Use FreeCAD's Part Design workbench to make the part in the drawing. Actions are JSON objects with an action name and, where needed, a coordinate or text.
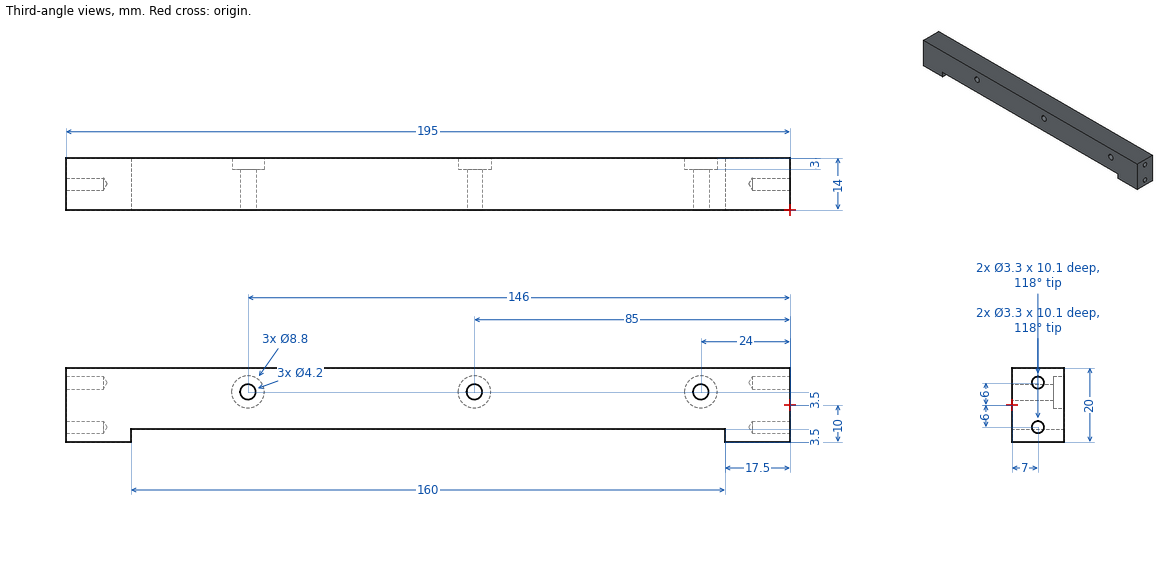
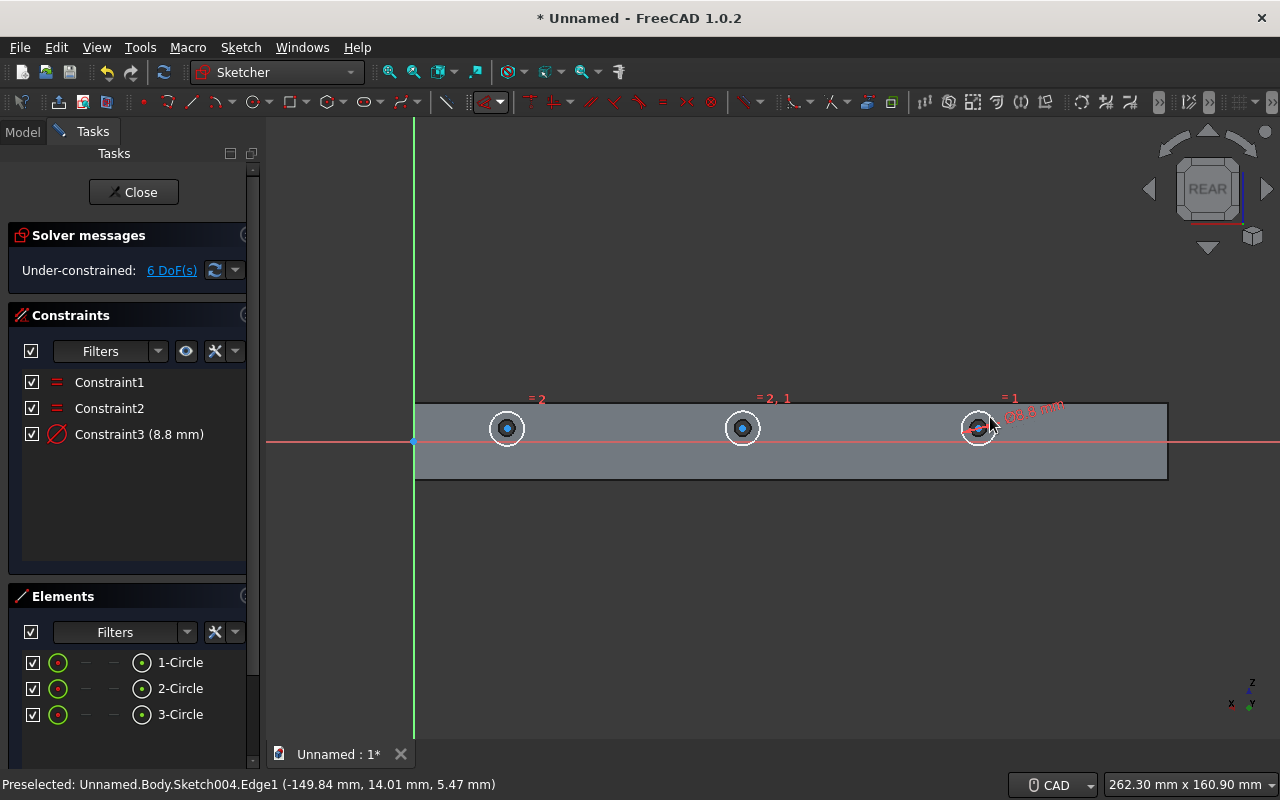
{"action": "left_click", "coordinate": [743, 428]}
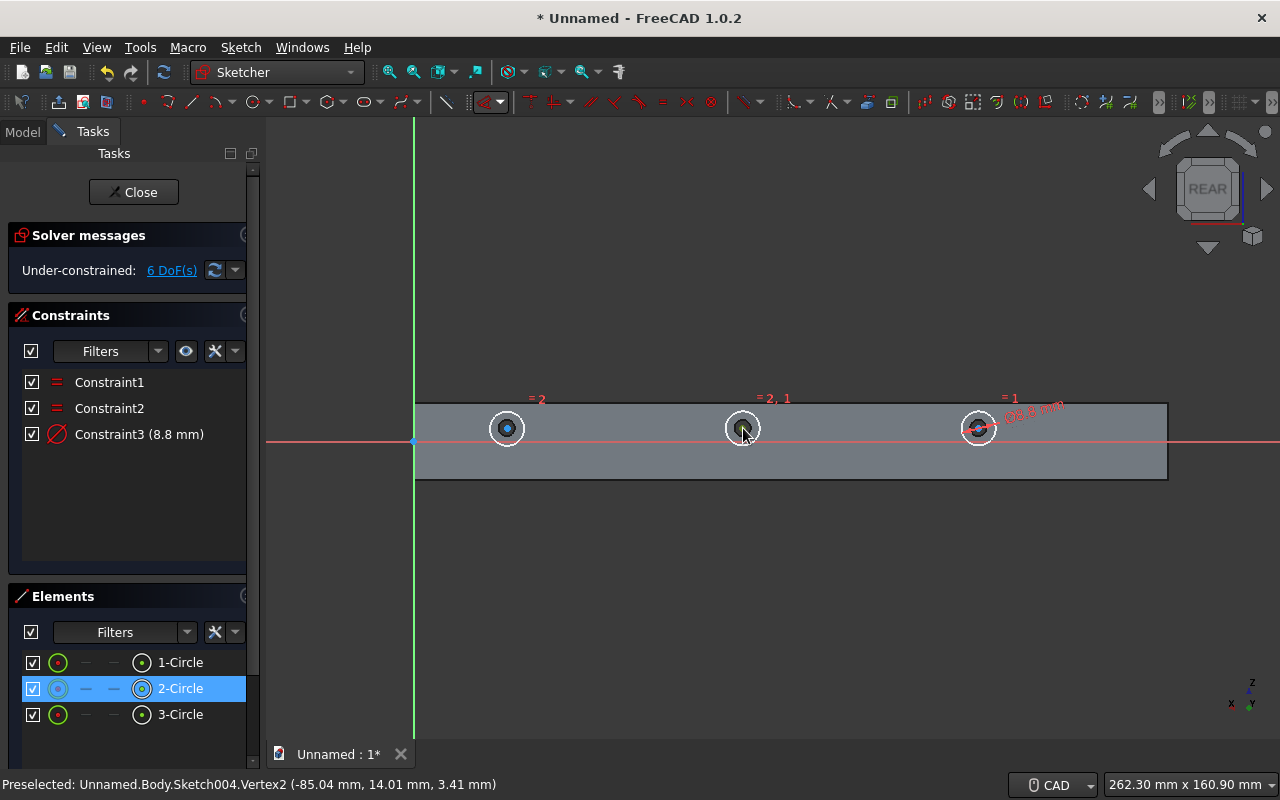
{"action": "key", "text": "l"}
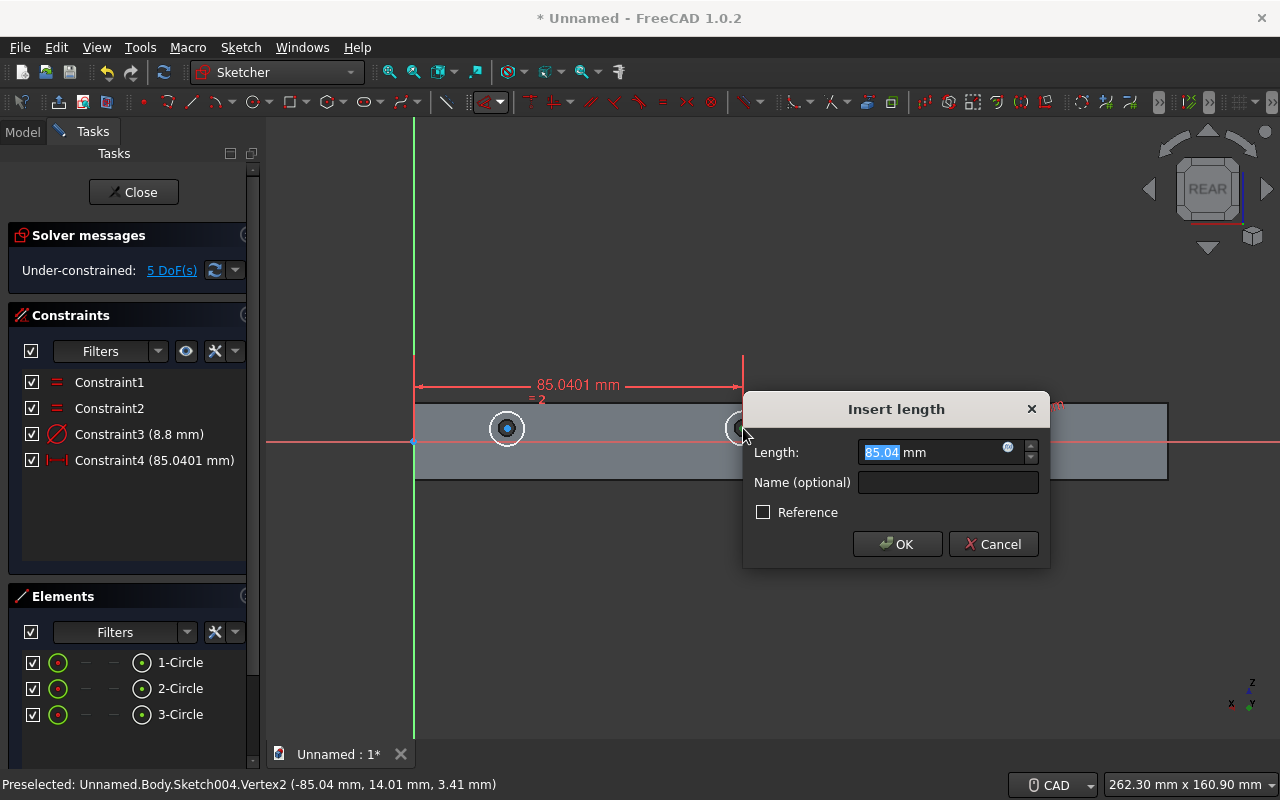
{"action": "type", "text": "85"}
{"action": "key", "text": "Return"}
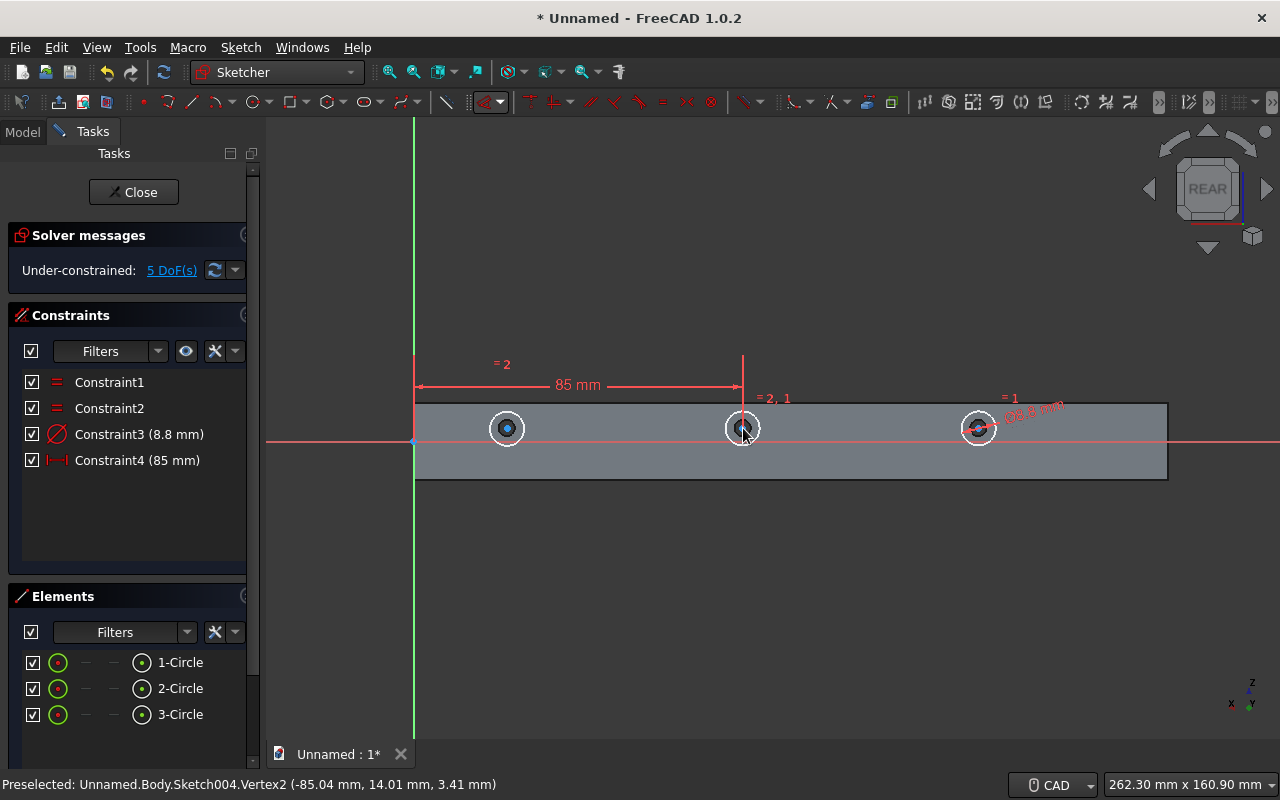
{"action": "left_click", "coordinate": [507, 429]}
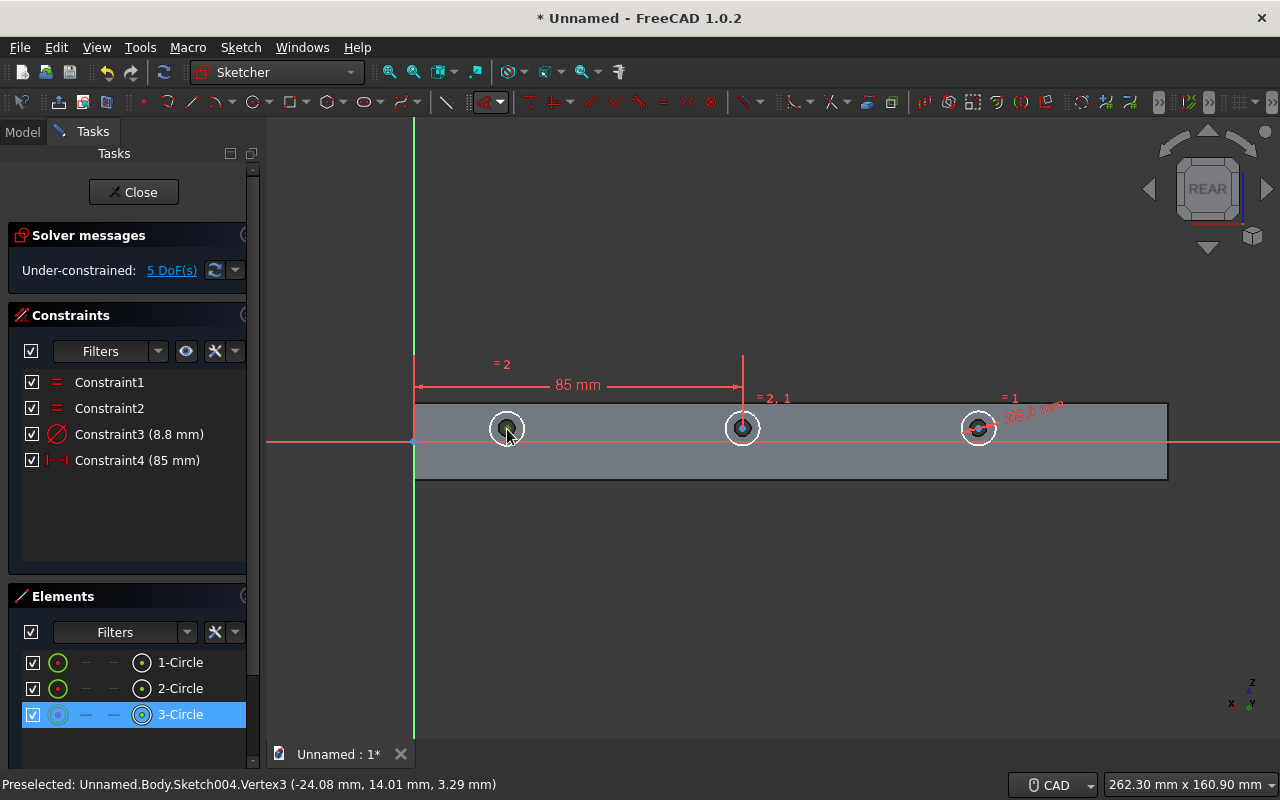
{"action": "key", "text": "l"}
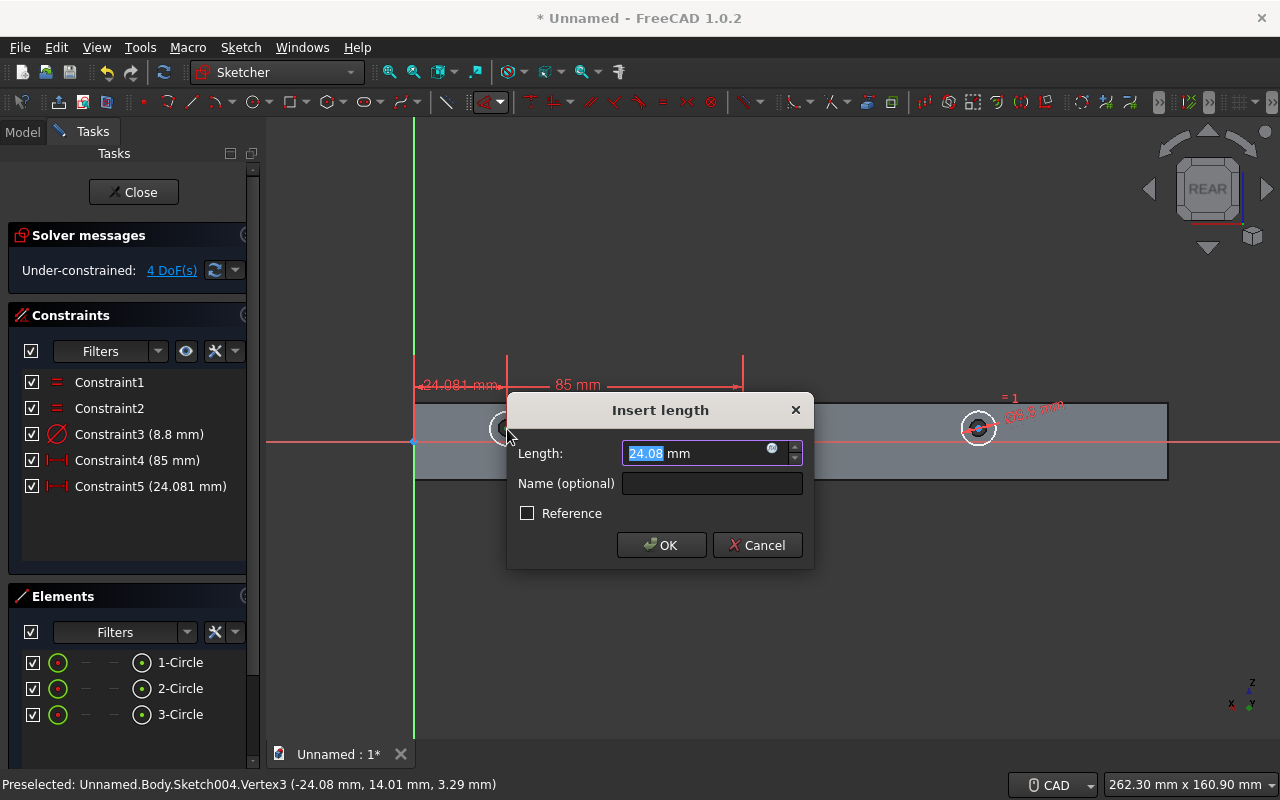
{"action": "type", "text": "24"}
{"action": "key", "text": "Return"}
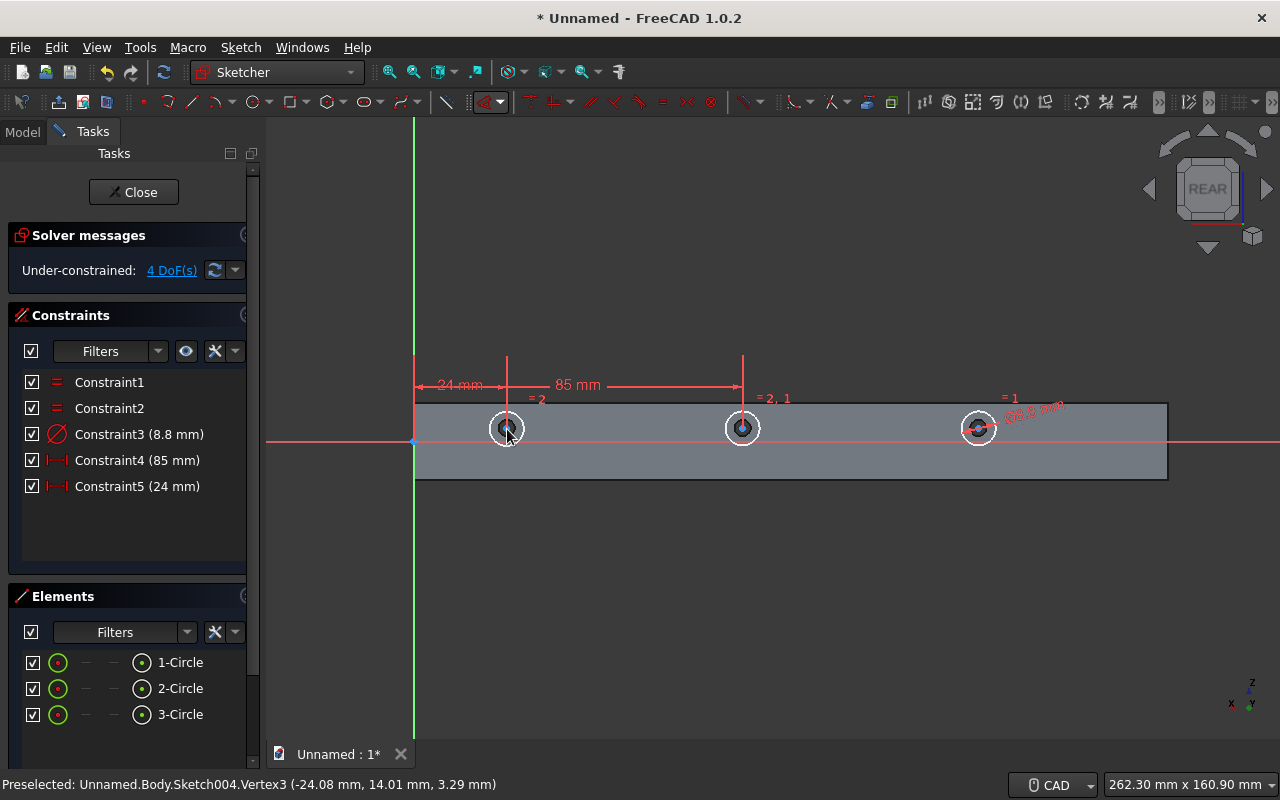
{"action": "left_click", "coordinate": [979, 428]}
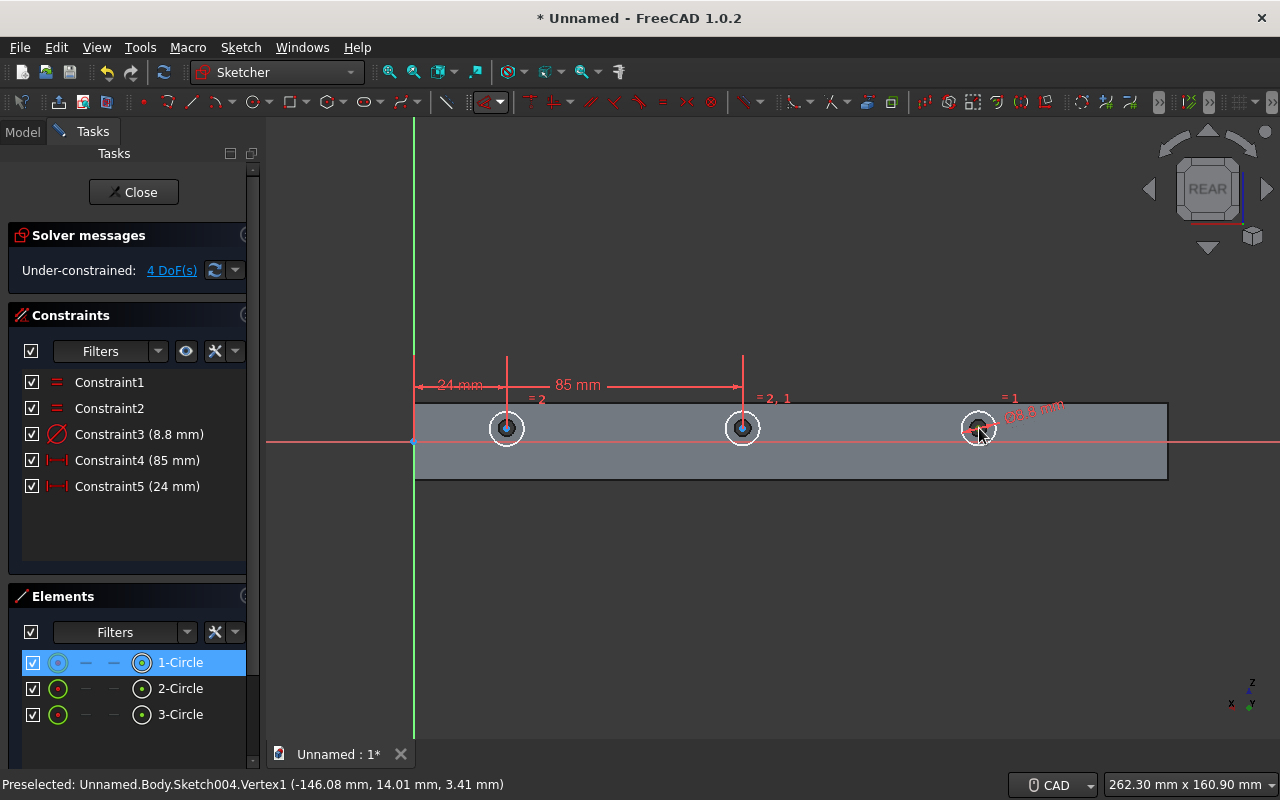
{"action": "key", "text": "l"}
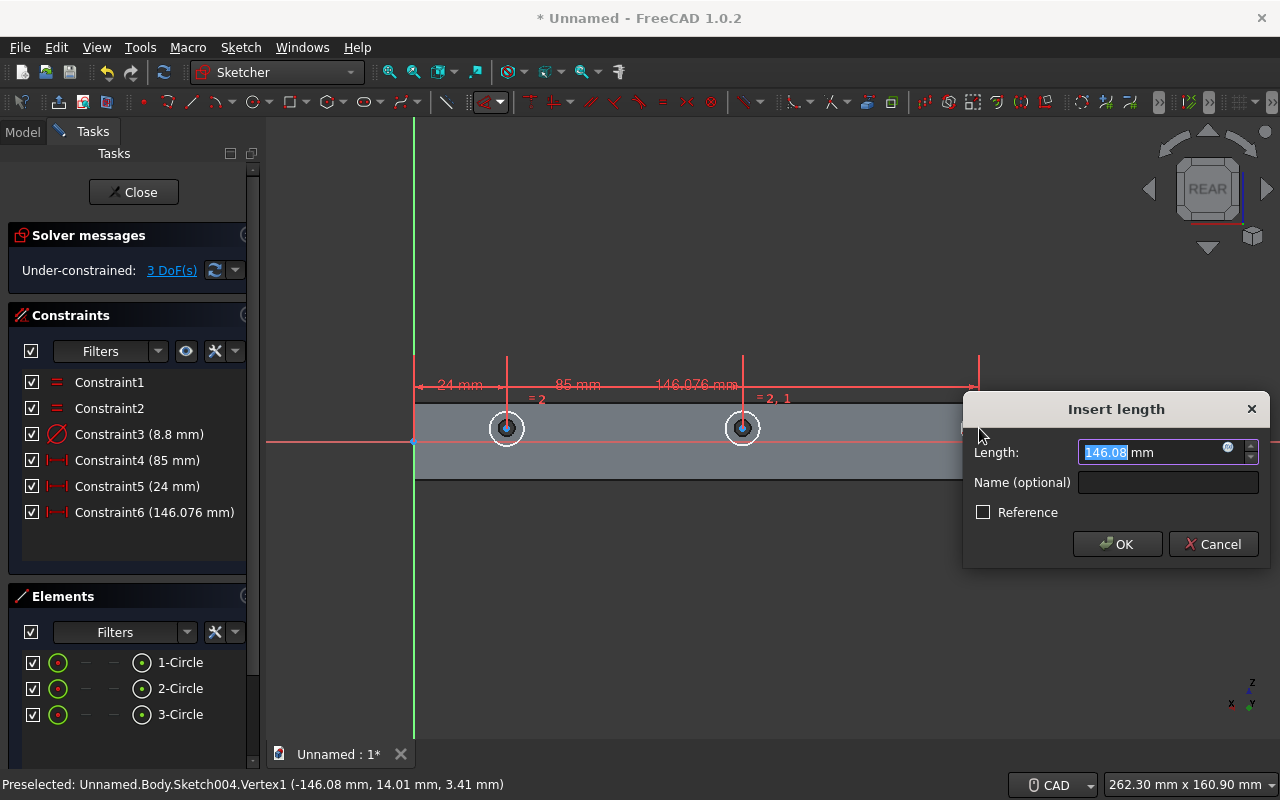
{"action": "type", "text": "146"}
{"action": "key", "text": "Return"}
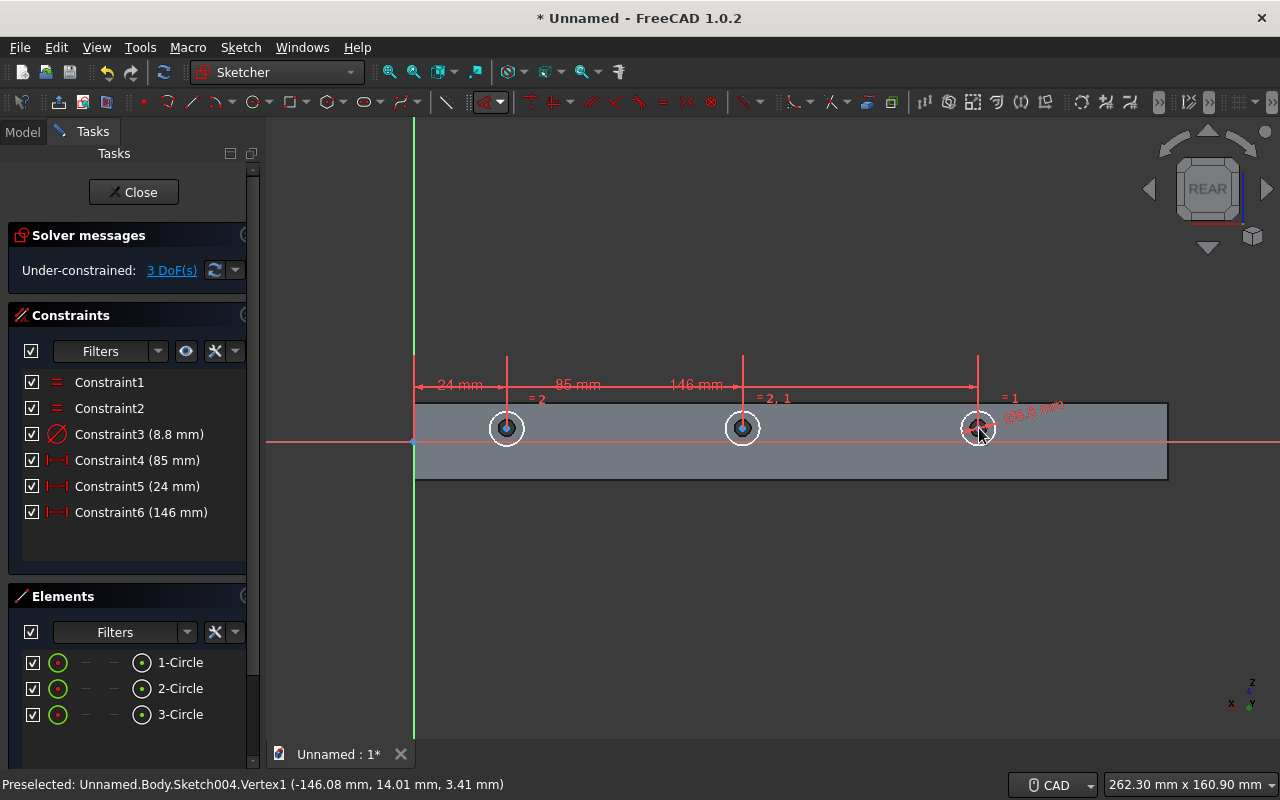
{"action": "scroll", "coordinate": [978, 428], "scroll_direction": "up", "scroll_amount": 6}